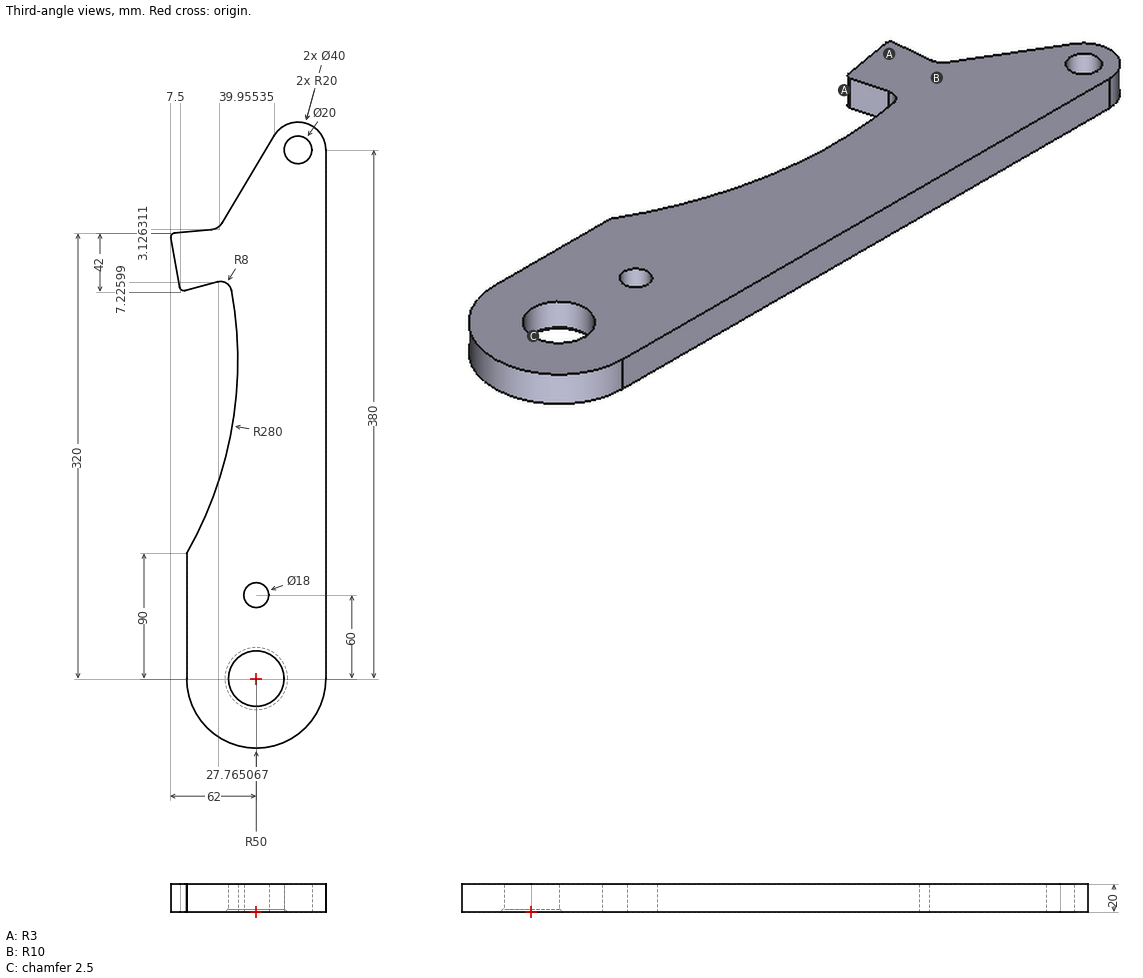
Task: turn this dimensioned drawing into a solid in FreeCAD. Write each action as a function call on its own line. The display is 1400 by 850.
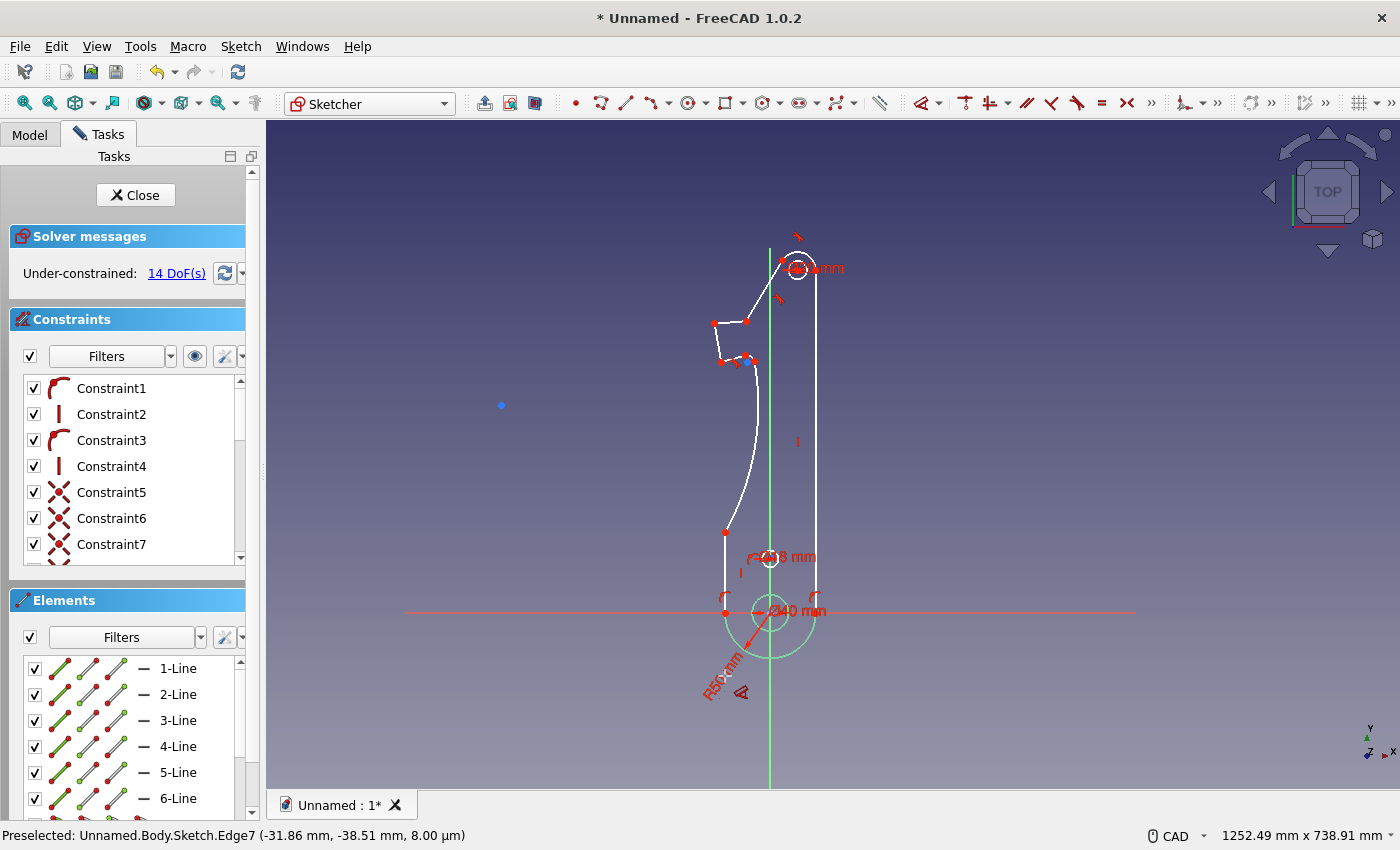
scroll(789, 254, up, 4)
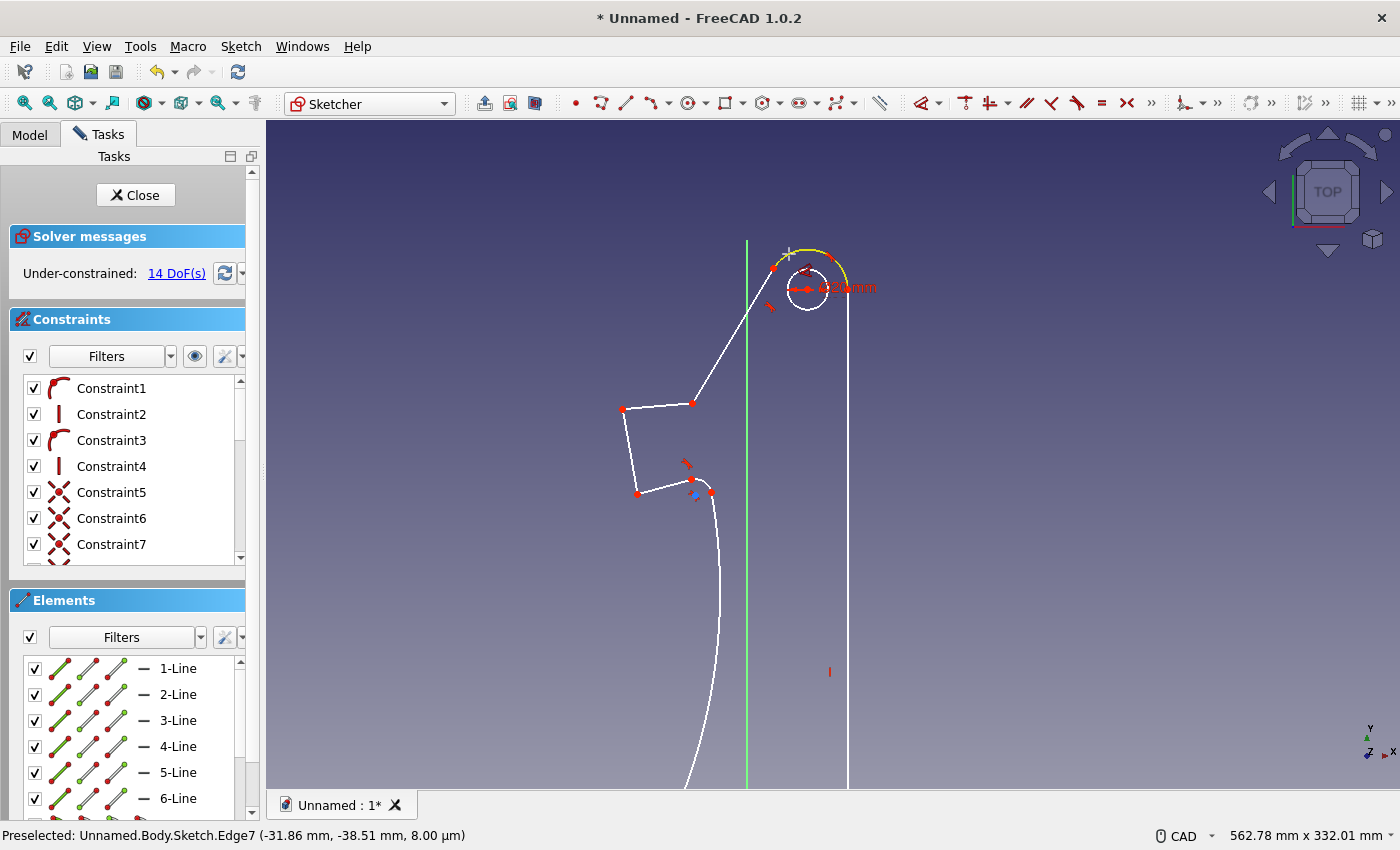
click(788, 255)
click(772, 227)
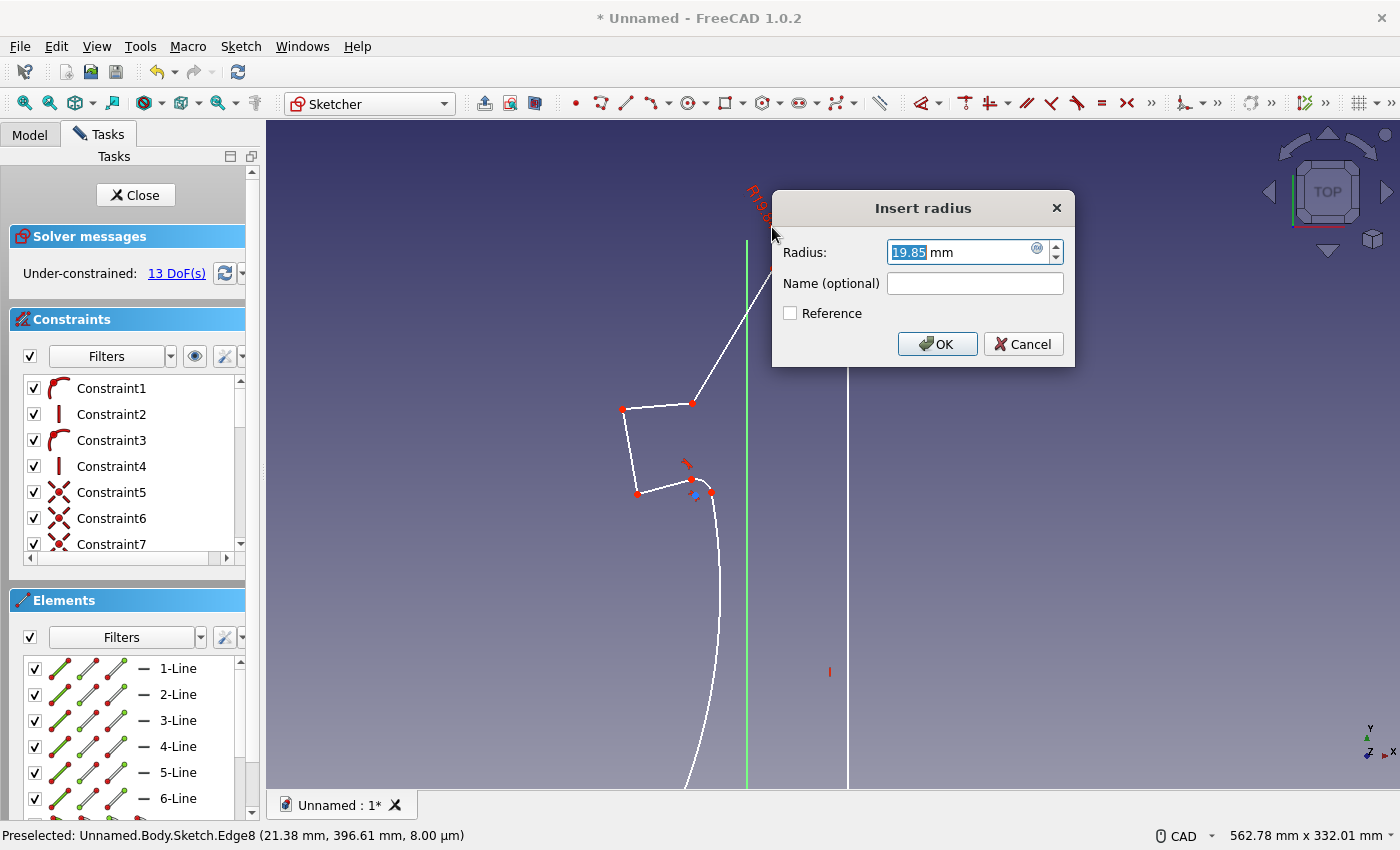
text(20)
key(Return)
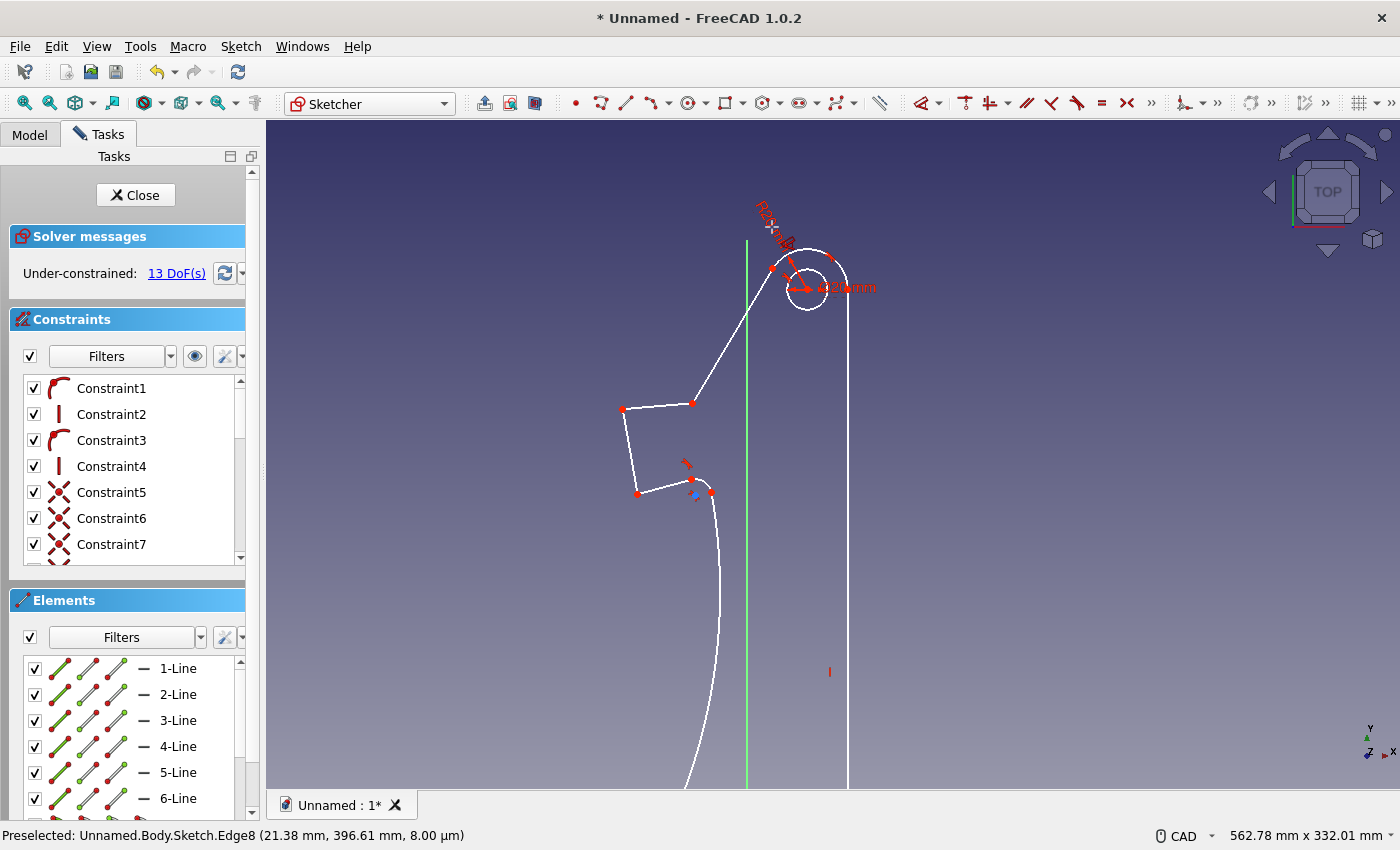
scroll(704, 482, up, 5)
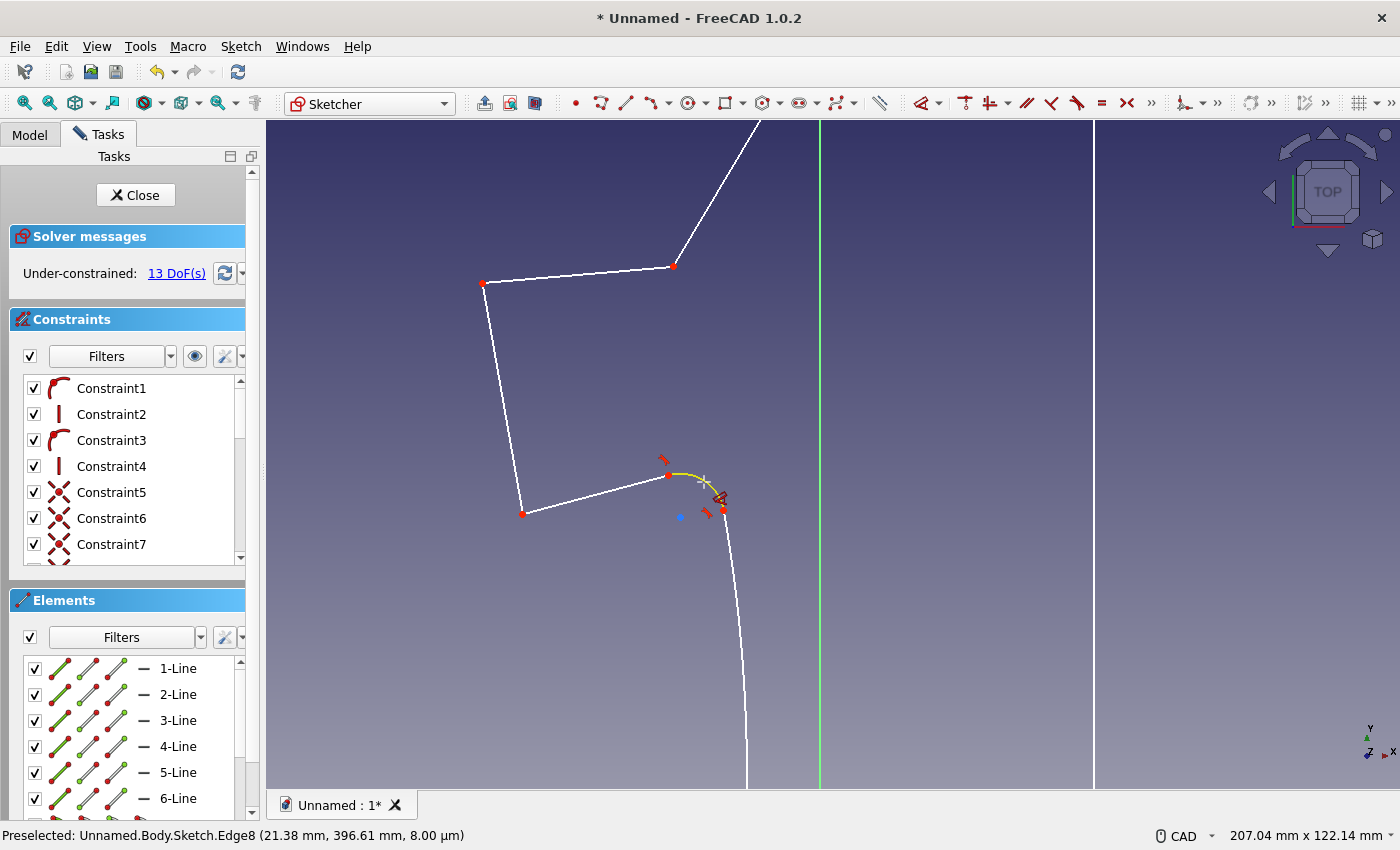
click(704, 481)
click(721, 454)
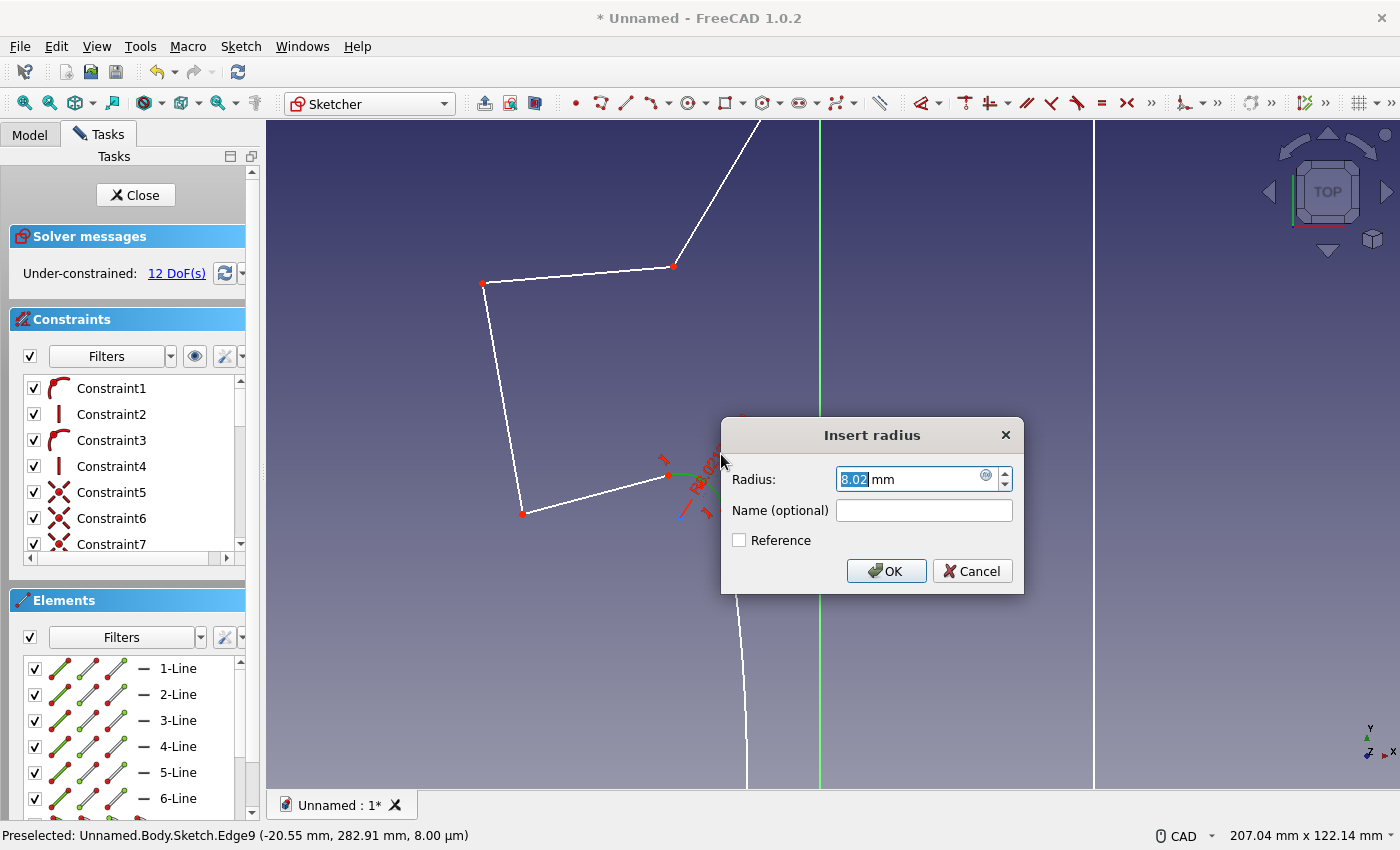
text(8)
key(Return)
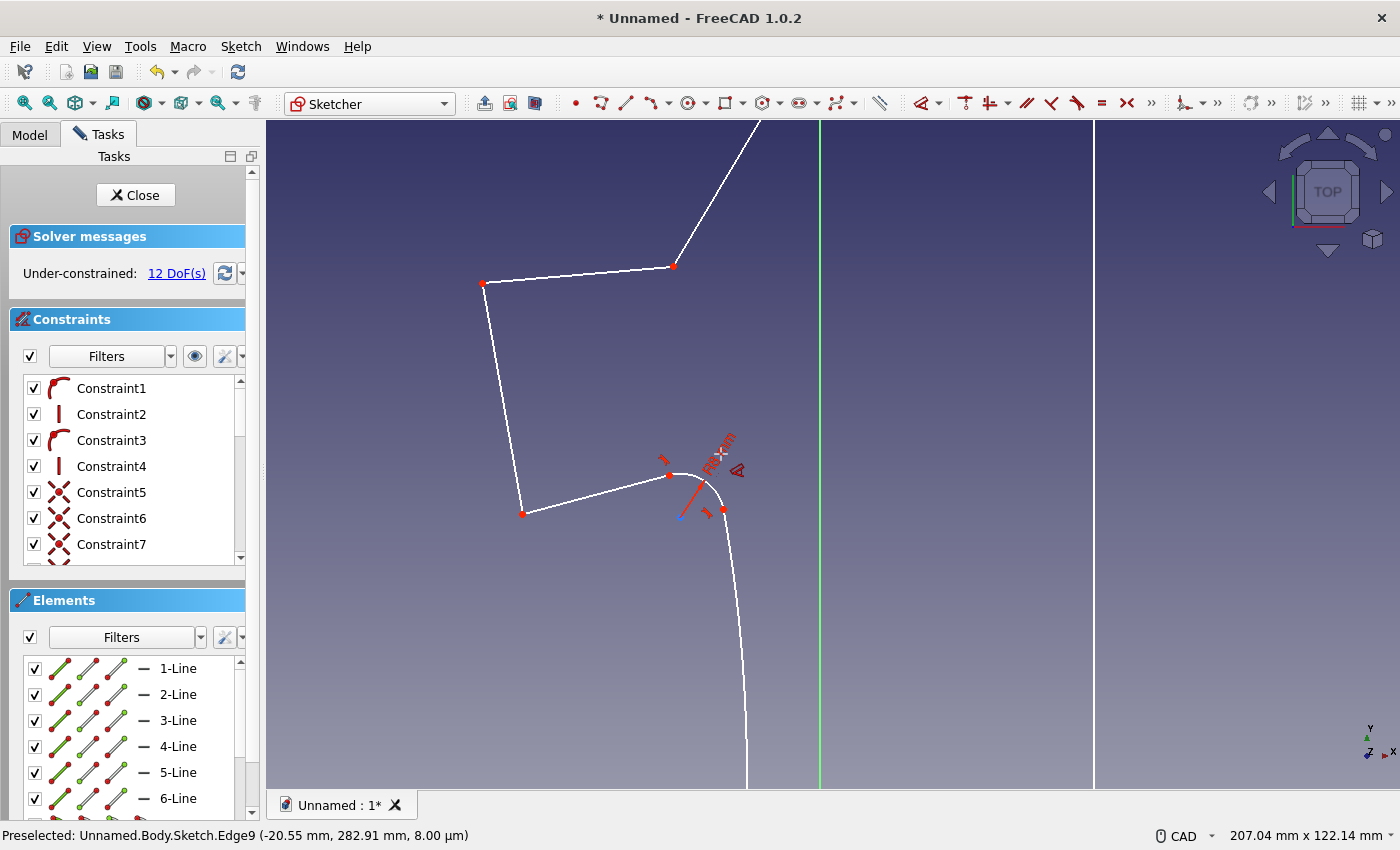
scroll(760, 331, down, 9)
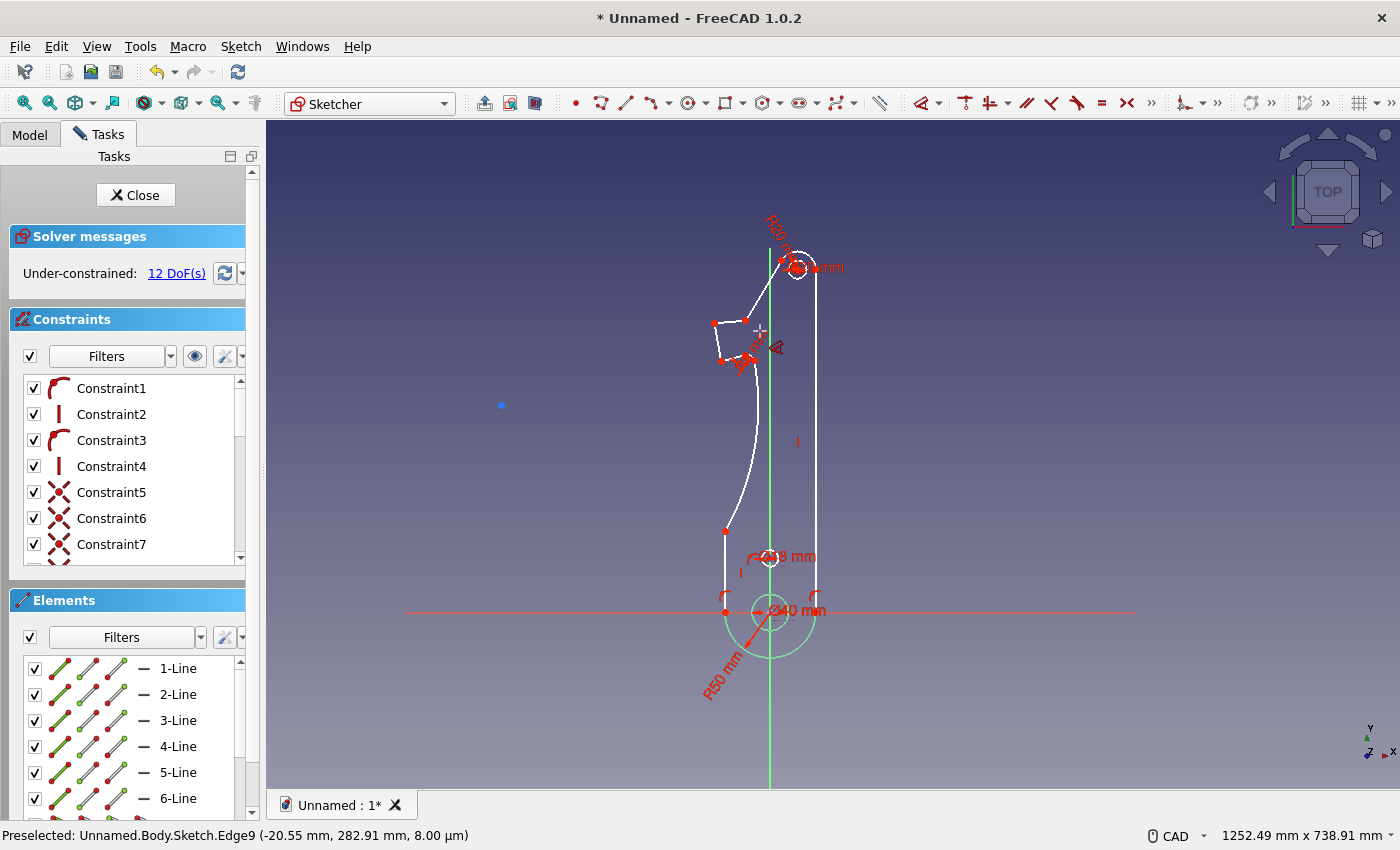
click(758, 396)
click(790, 395)